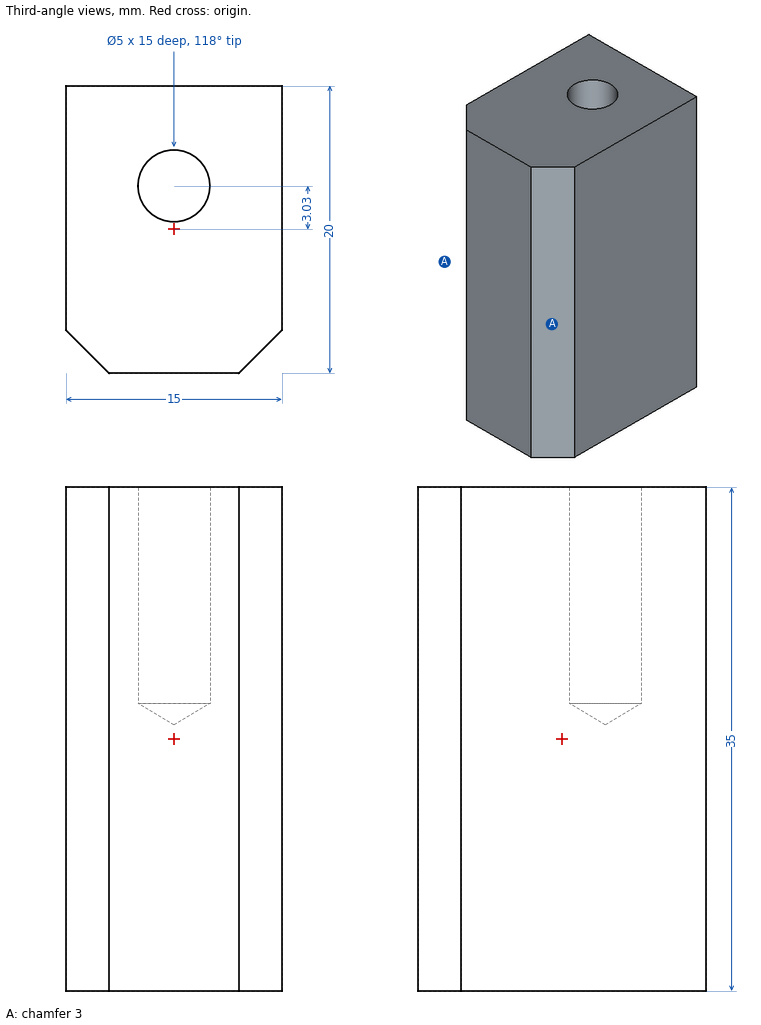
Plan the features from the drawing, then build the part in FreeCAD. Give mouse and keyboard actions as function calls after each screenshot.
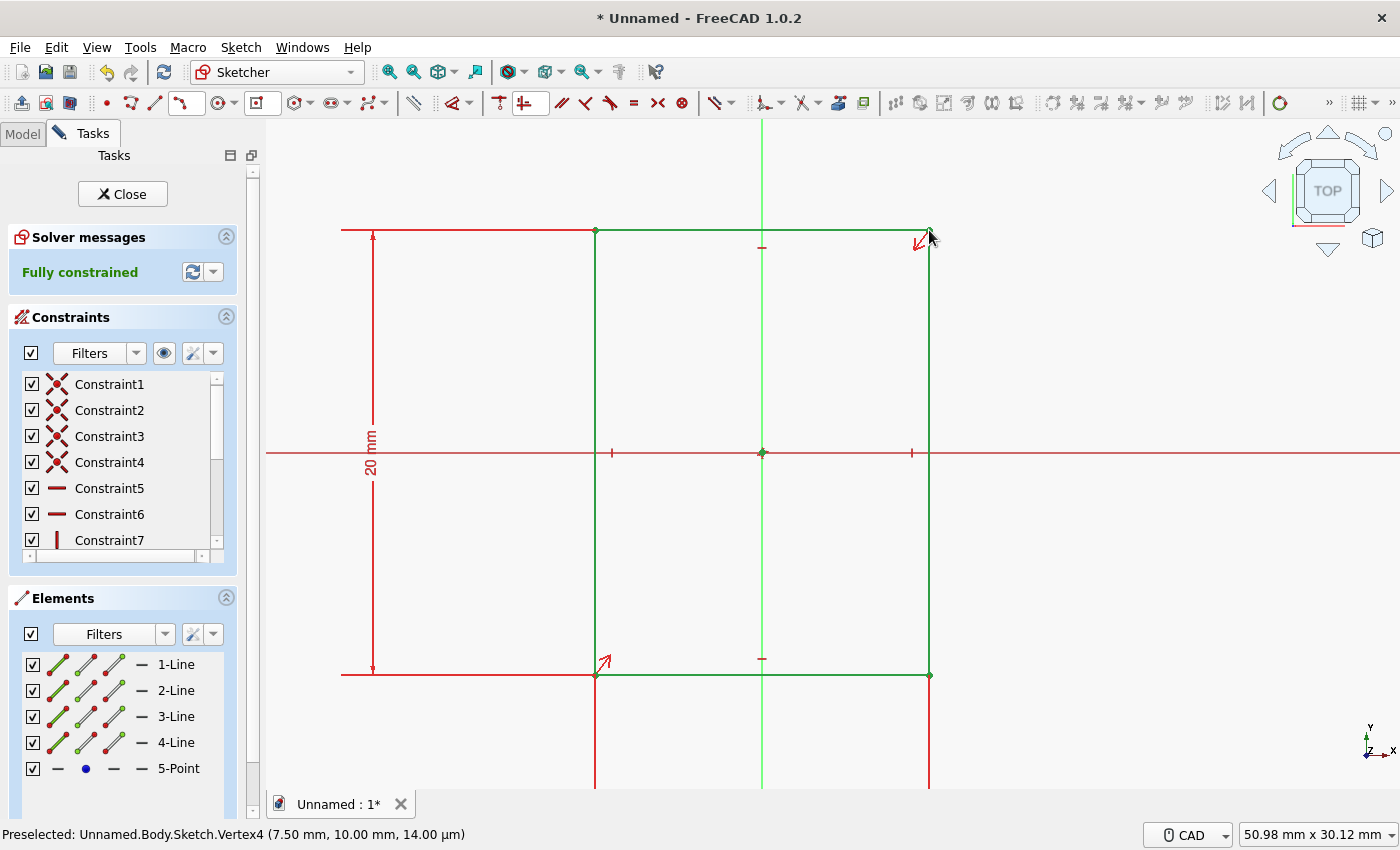
click(123, 194)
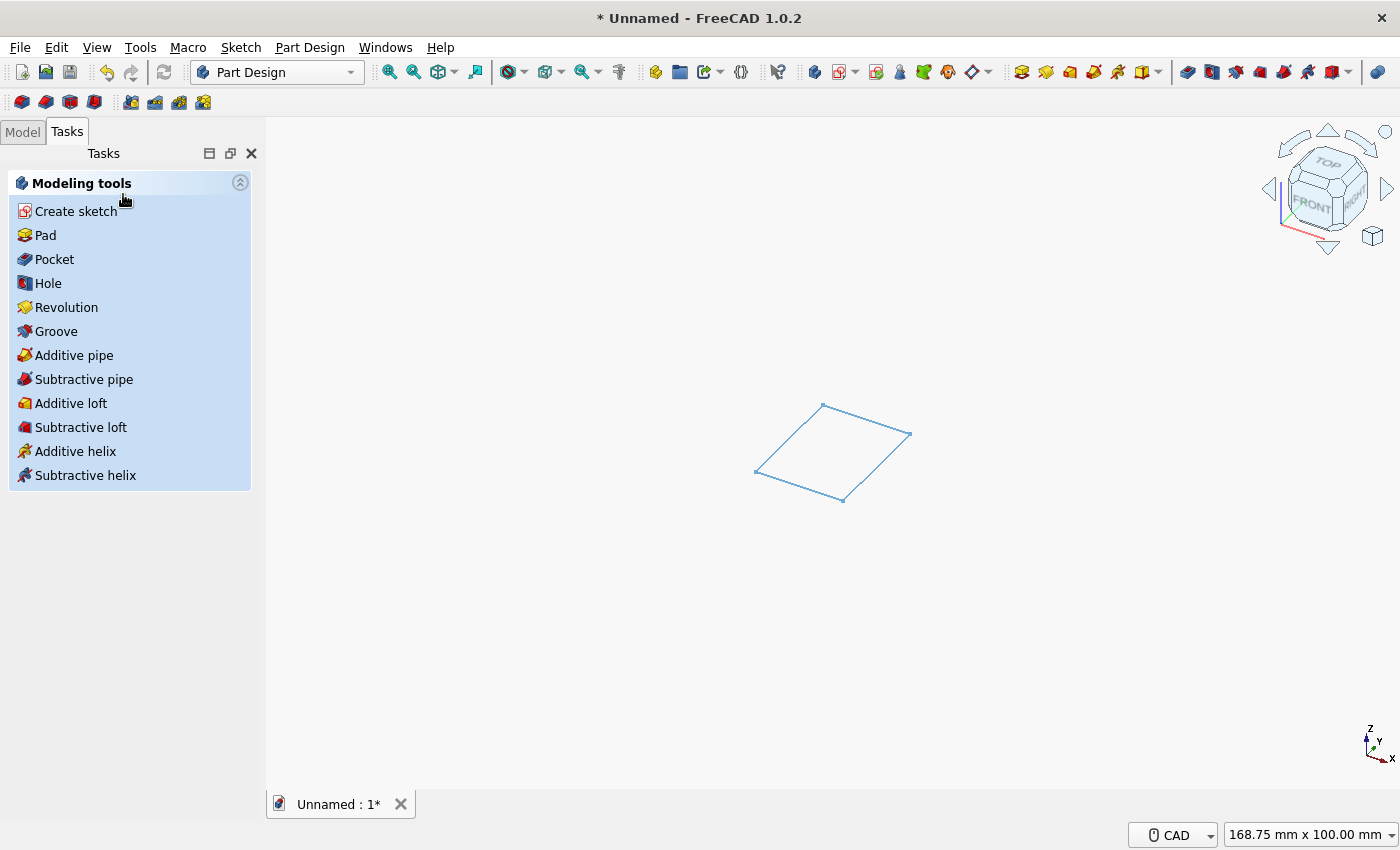
click(1022, 72)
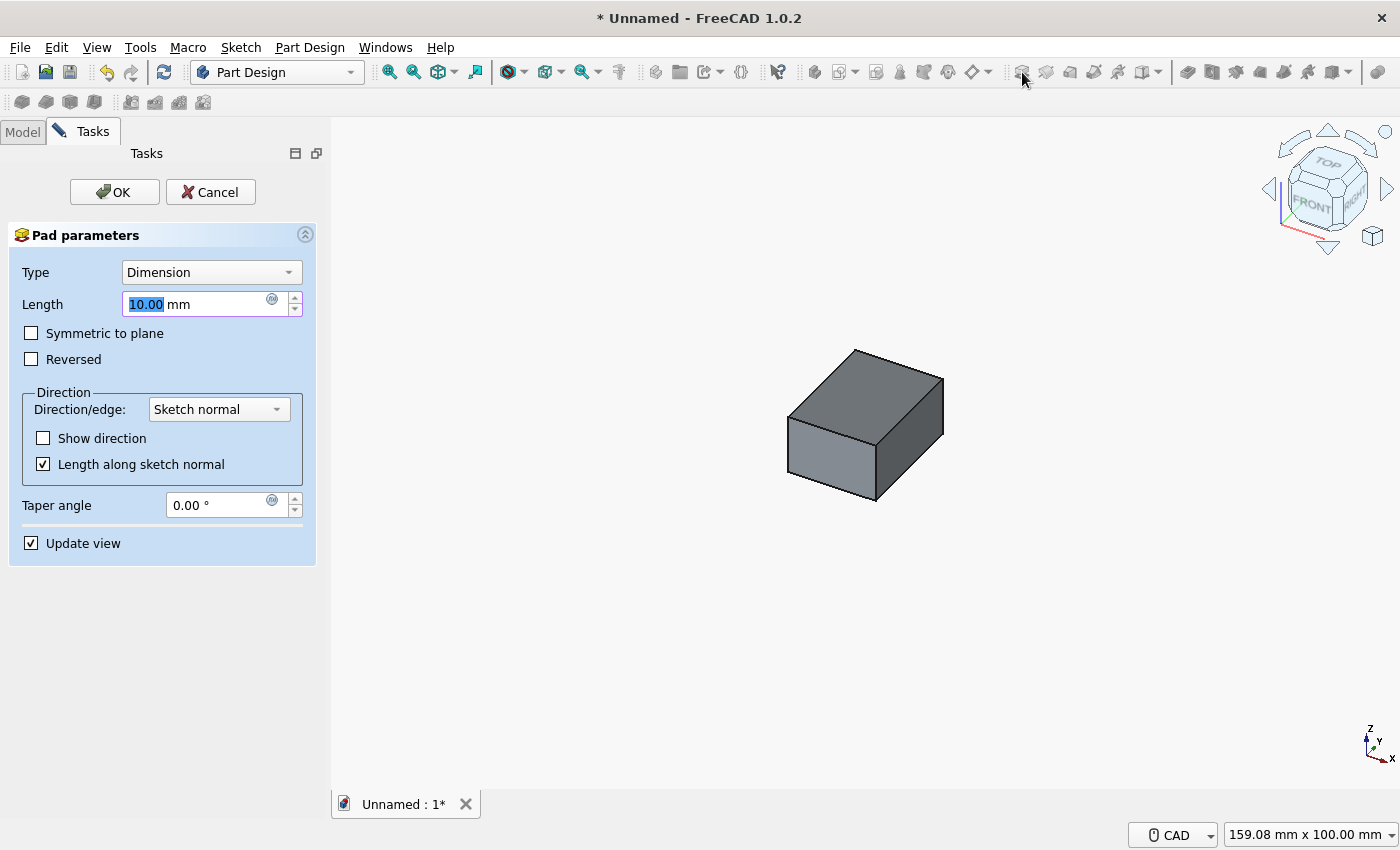
text(35)
key(Tab)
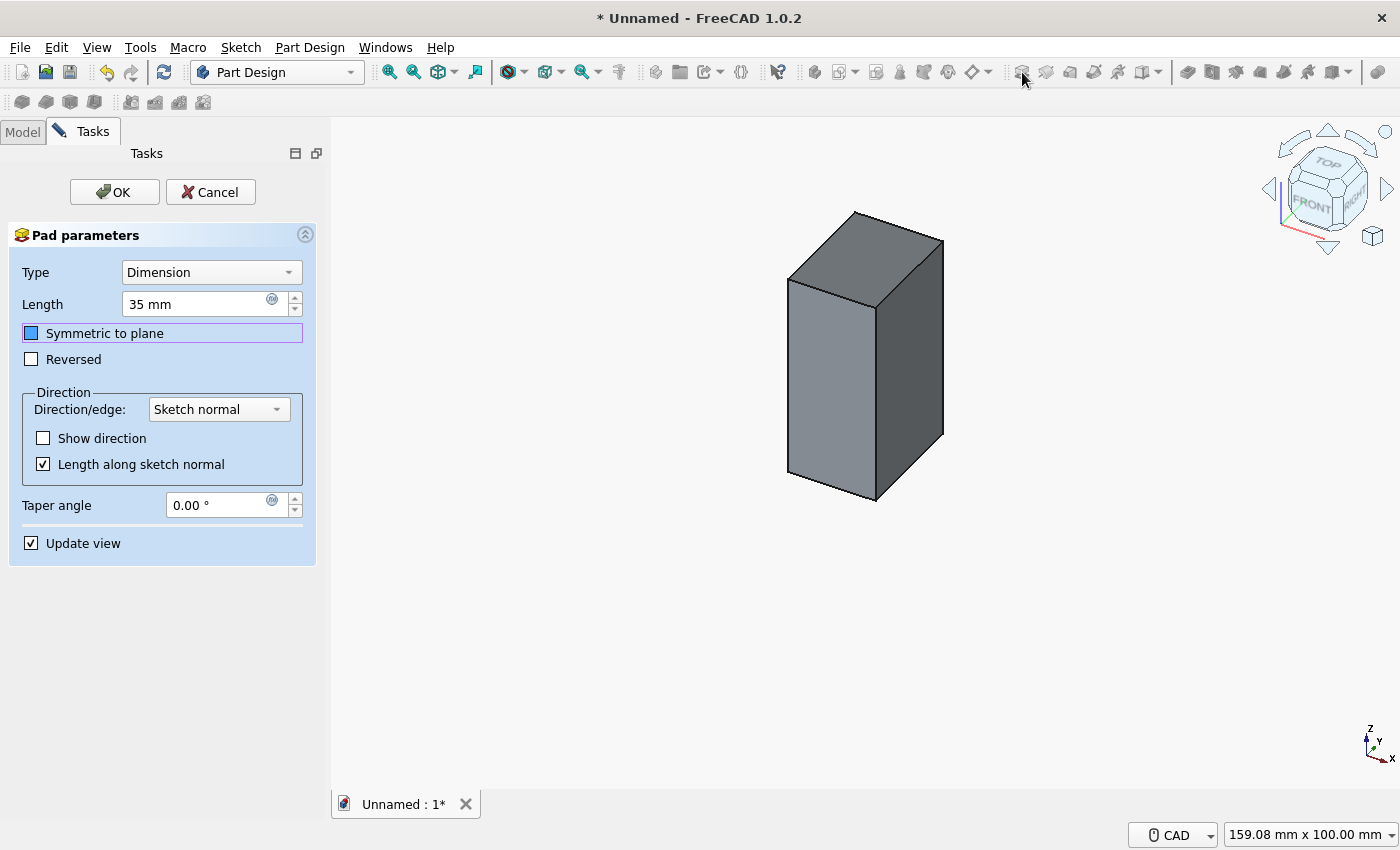
click(30, 333)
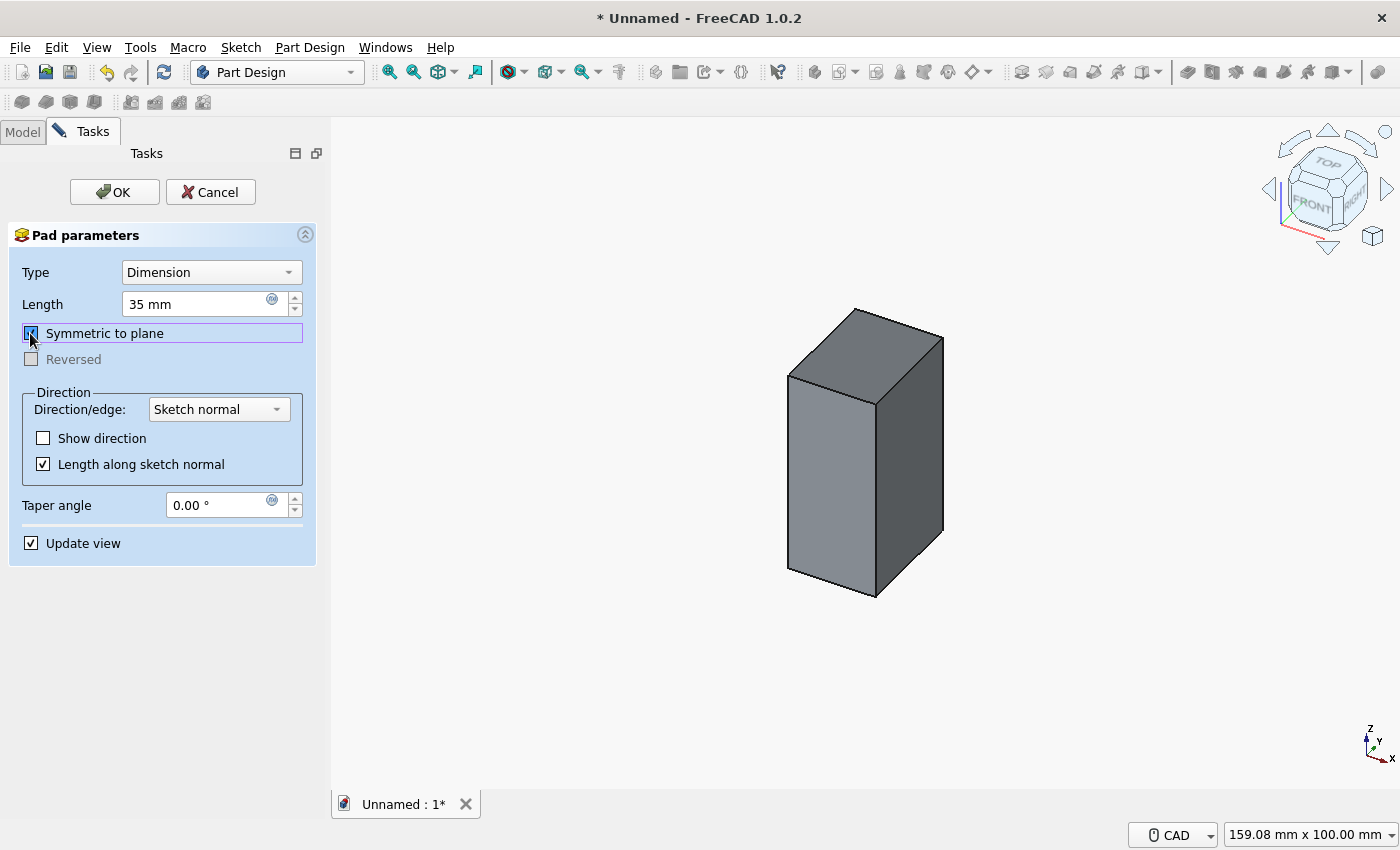
click(115, 192)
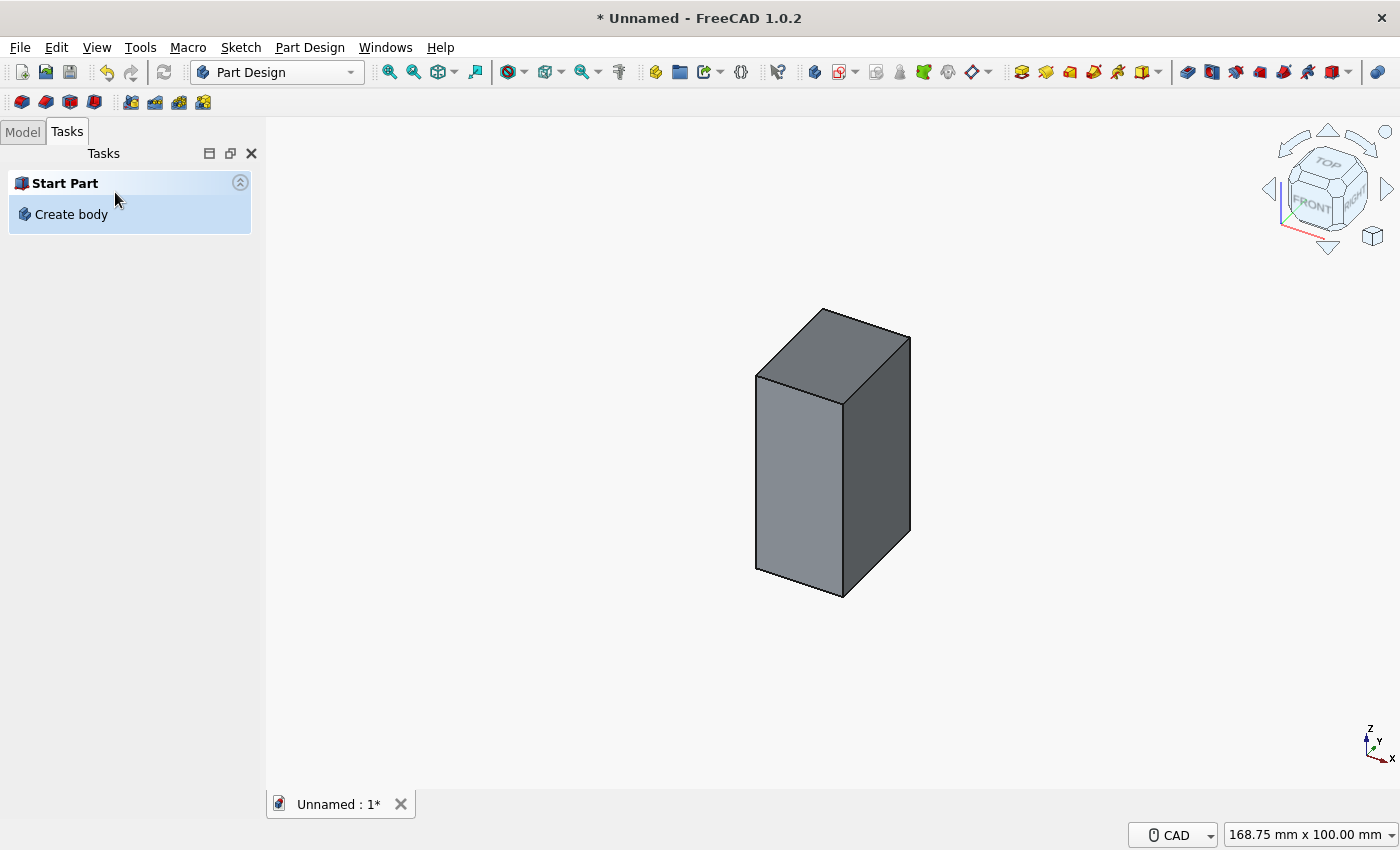
click(390, 72)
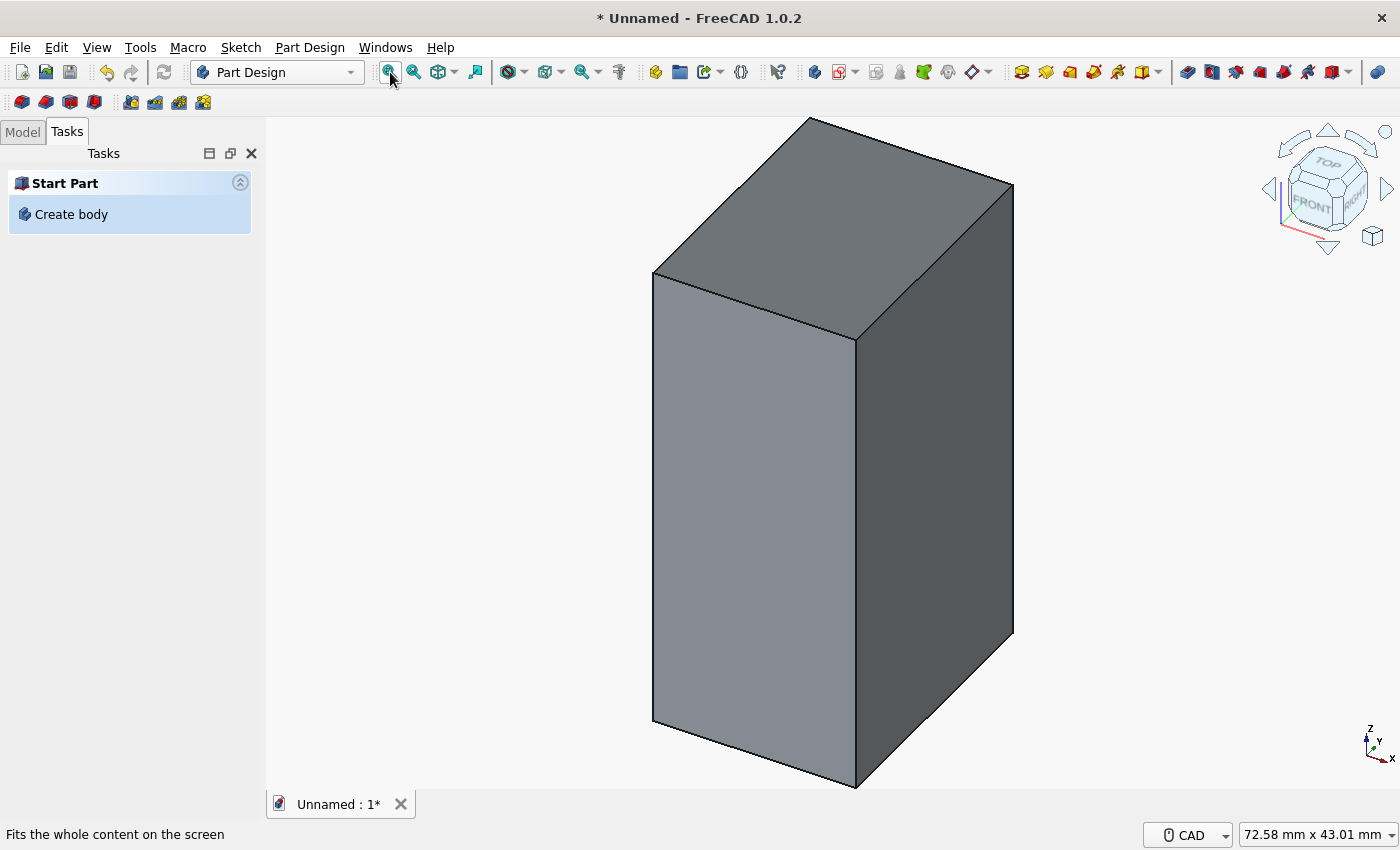
click(856, 563)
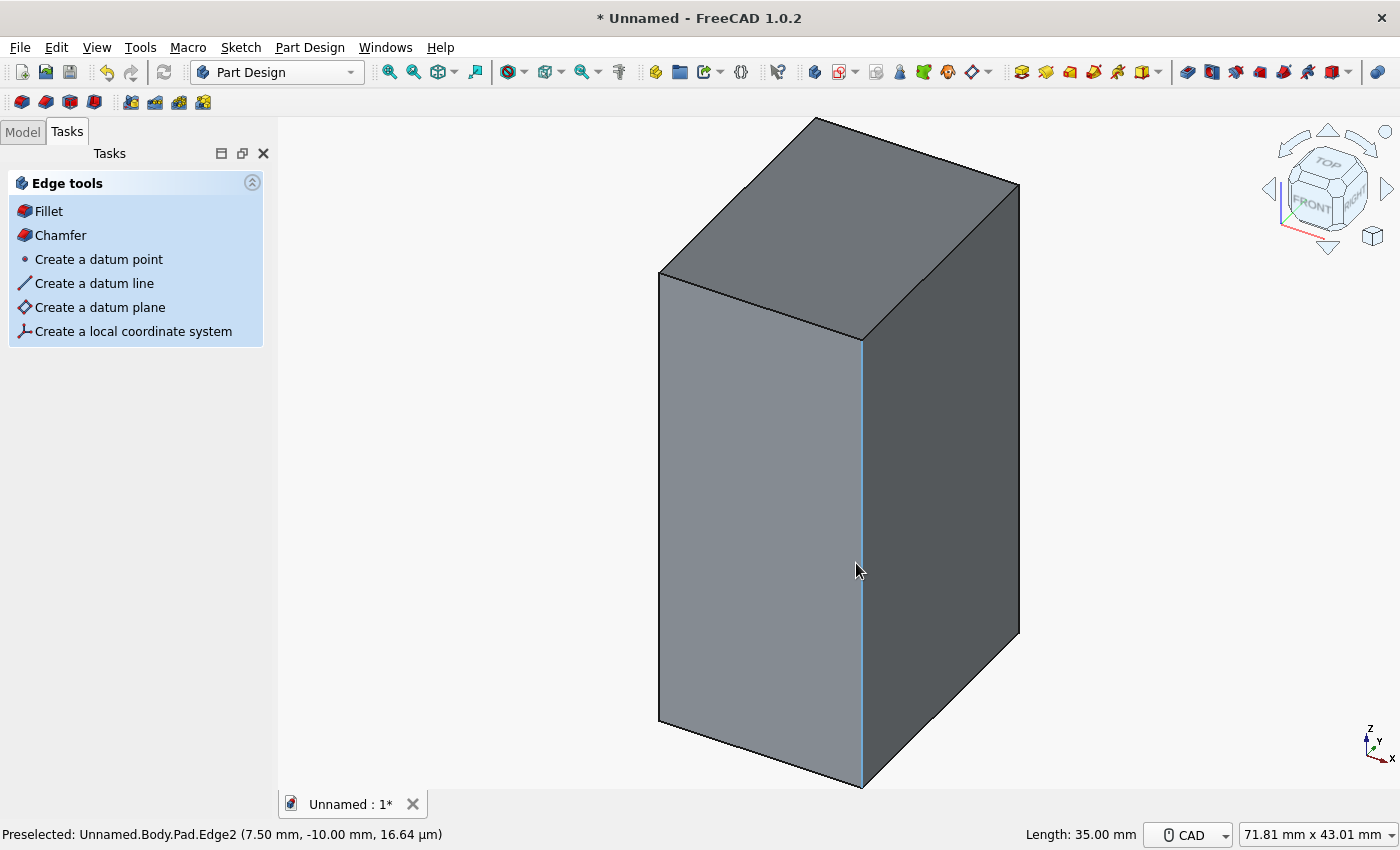
key(0)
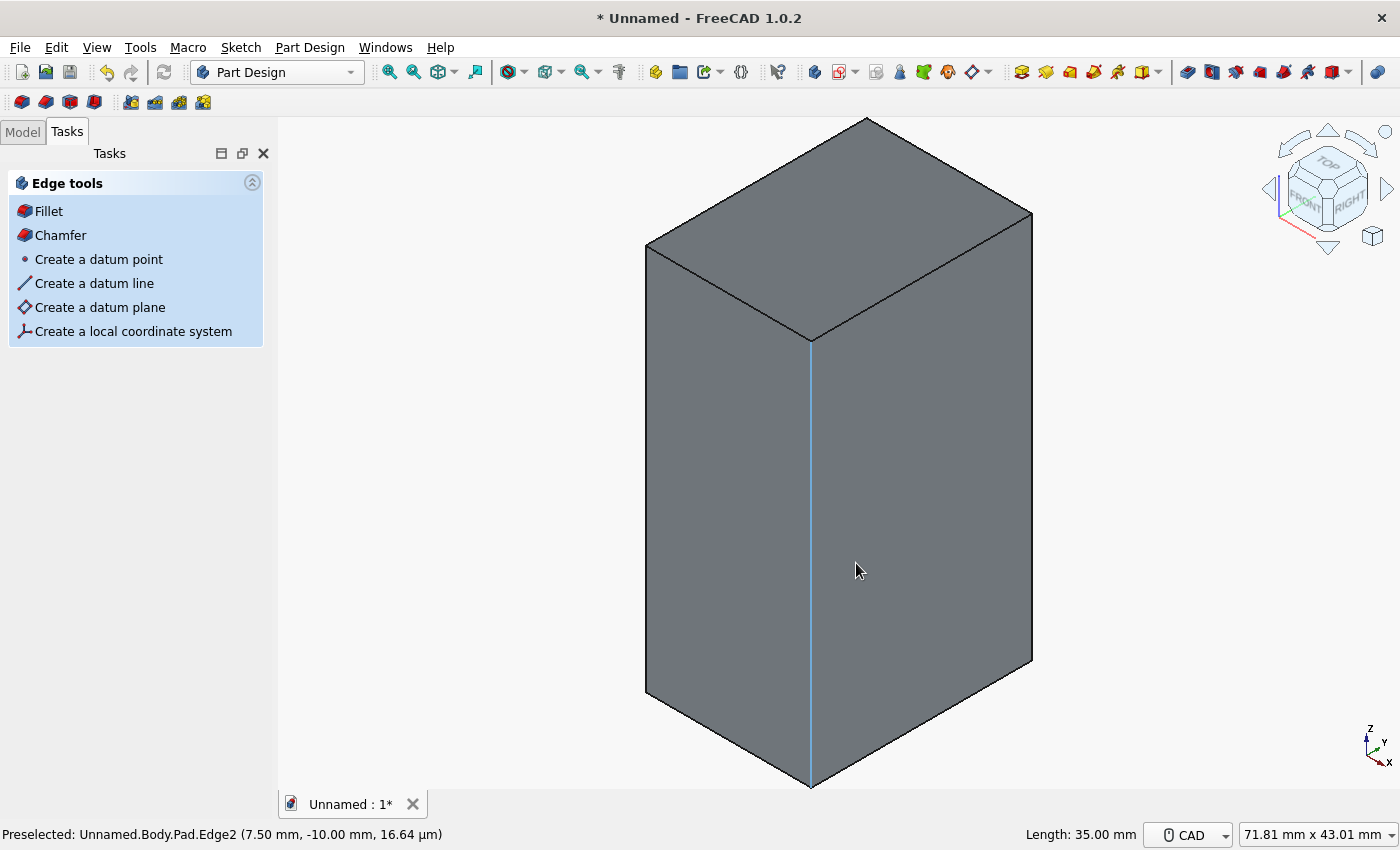
key(2)